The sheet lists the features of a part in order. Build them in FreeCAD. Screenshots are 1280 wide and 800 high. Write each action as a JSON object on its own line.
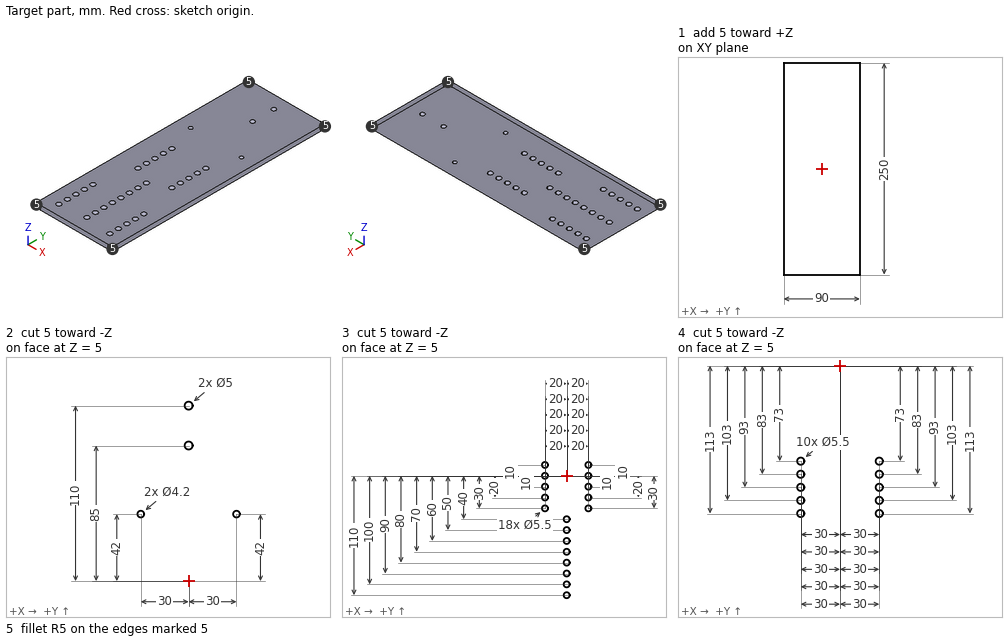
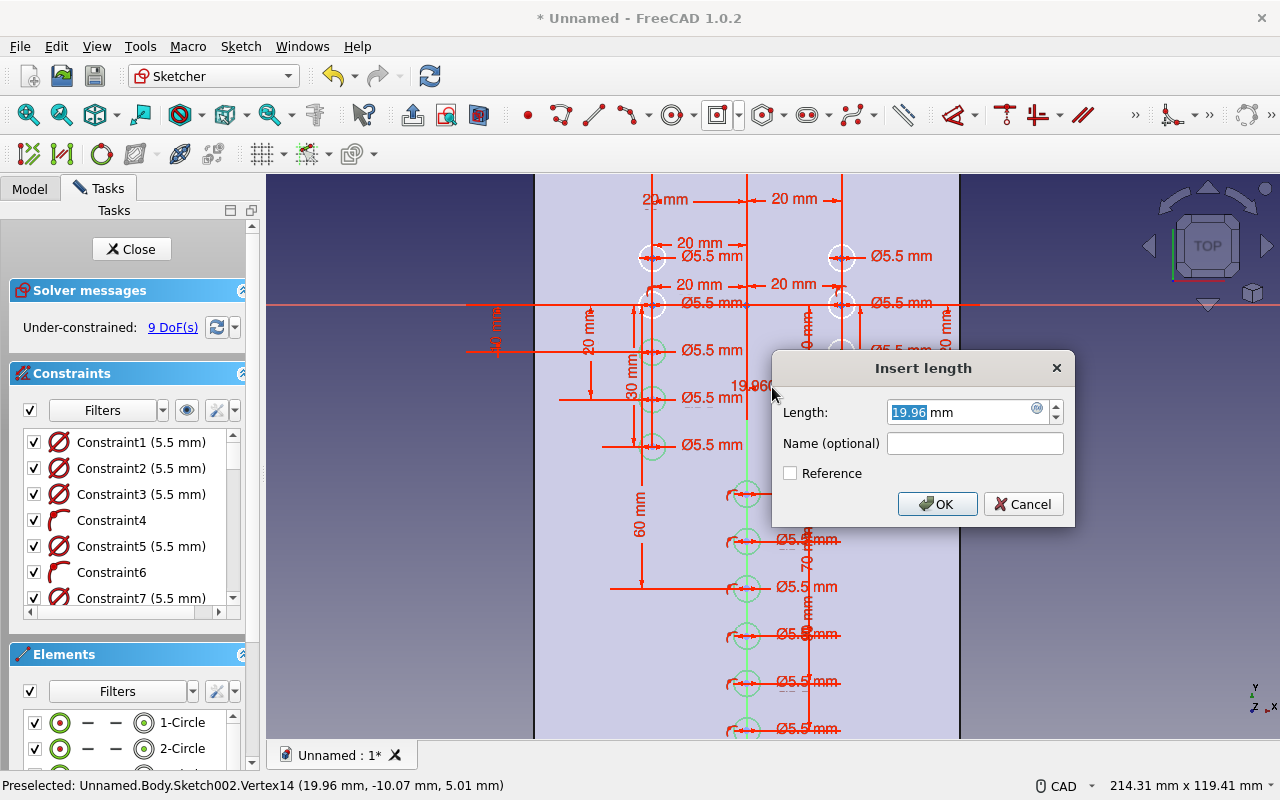
{"action": "type", "text": "20"}
{"action": "key", "text": "Return"}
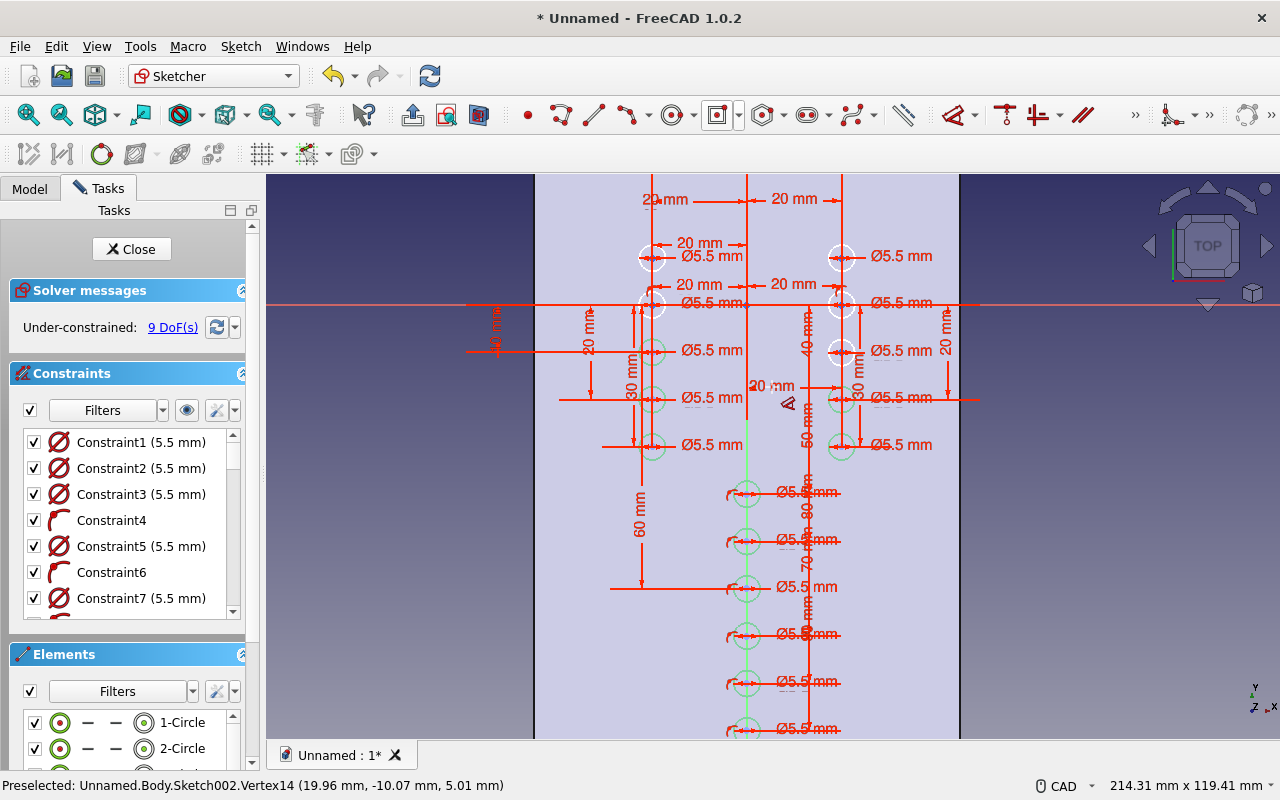
{"action": "left_click", "coordinate": [842, 353]}
{"action": "left_click", "coordinate": [713, 329]}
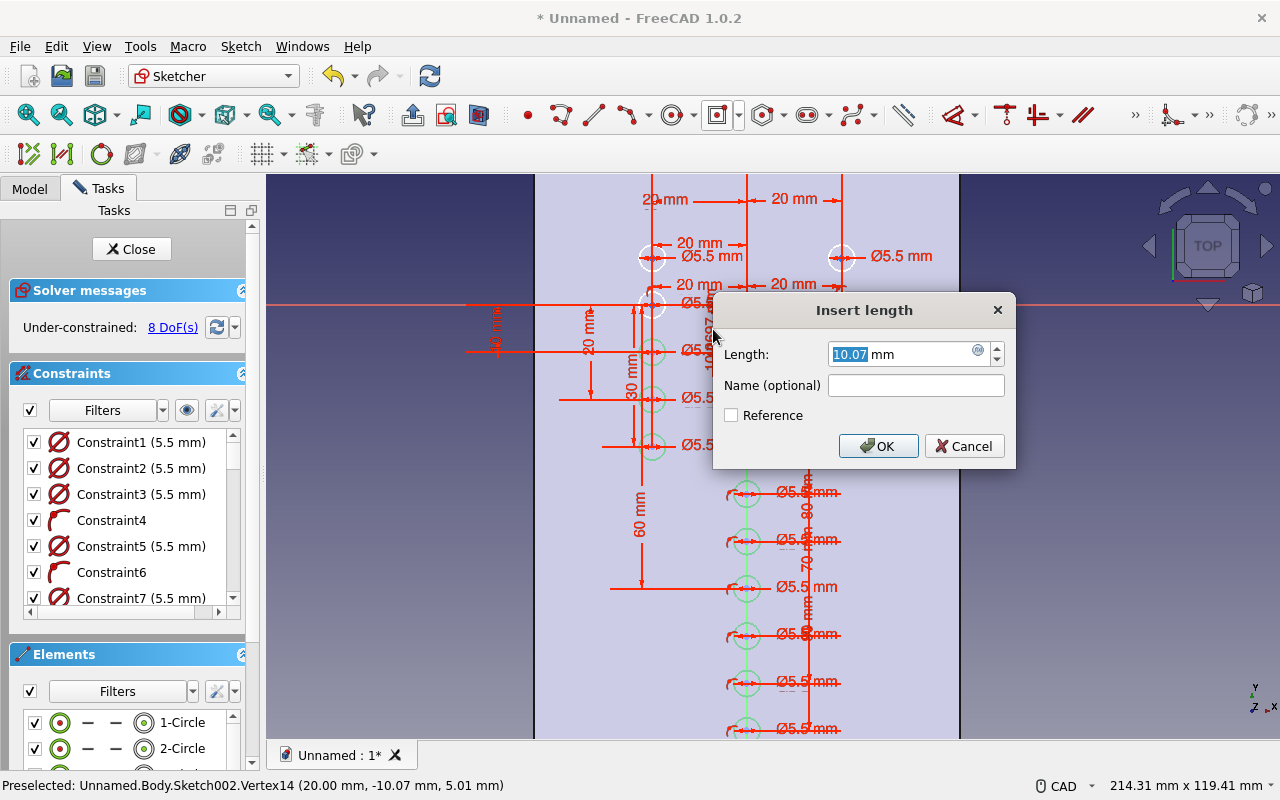
{"action": "type", "text": "10"}
{"action": "key", "text": "Return"}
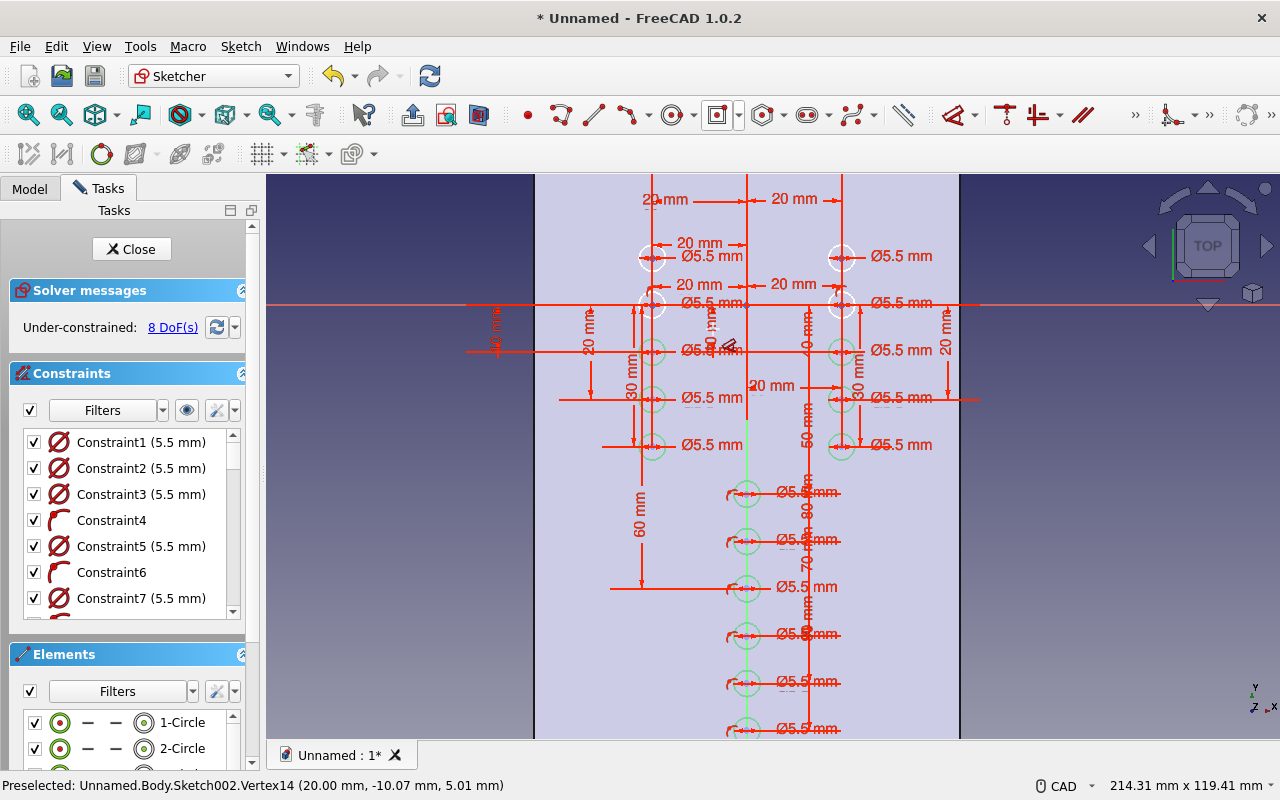
{"action": "left_click", "coordinate": [652, 305]}
{"action": "left_click", "coordinate": [721, 363]}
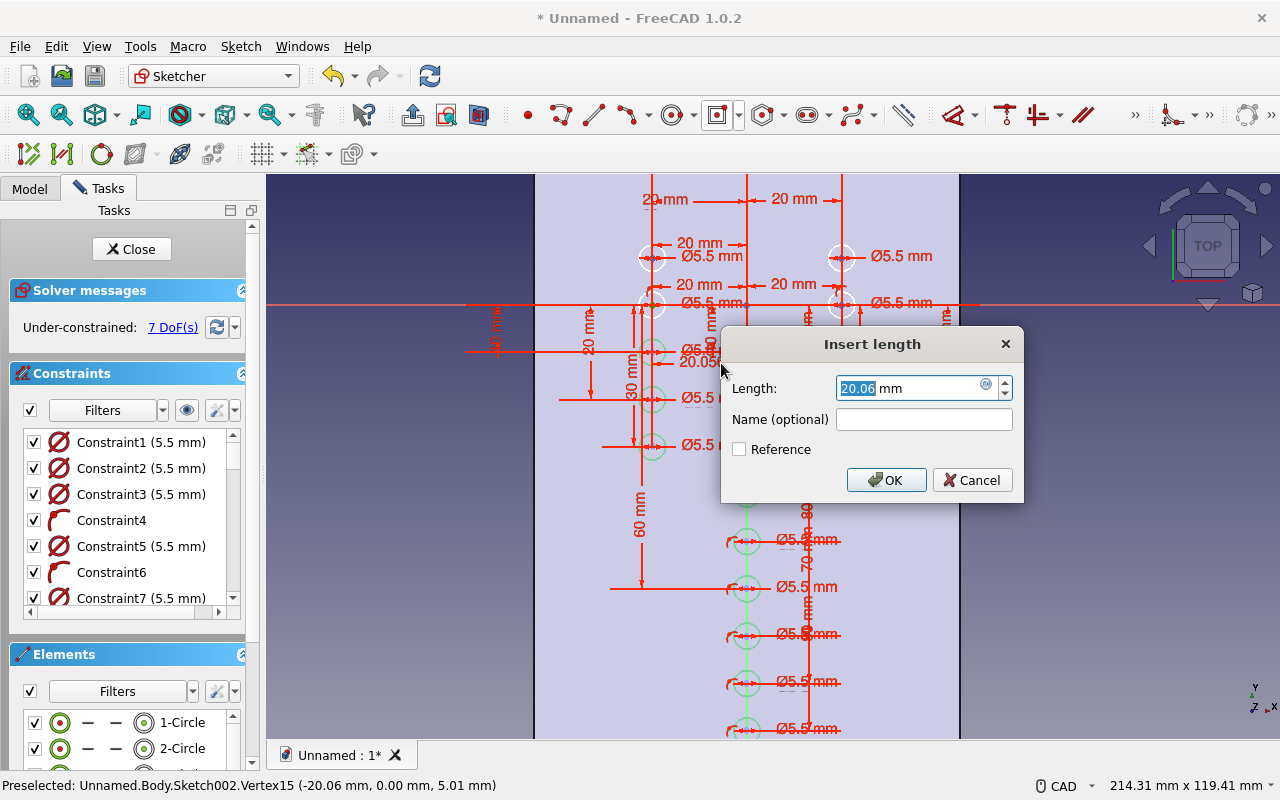
{"action": "type", "text": "20"}
{"action": "key", "text": "Return"}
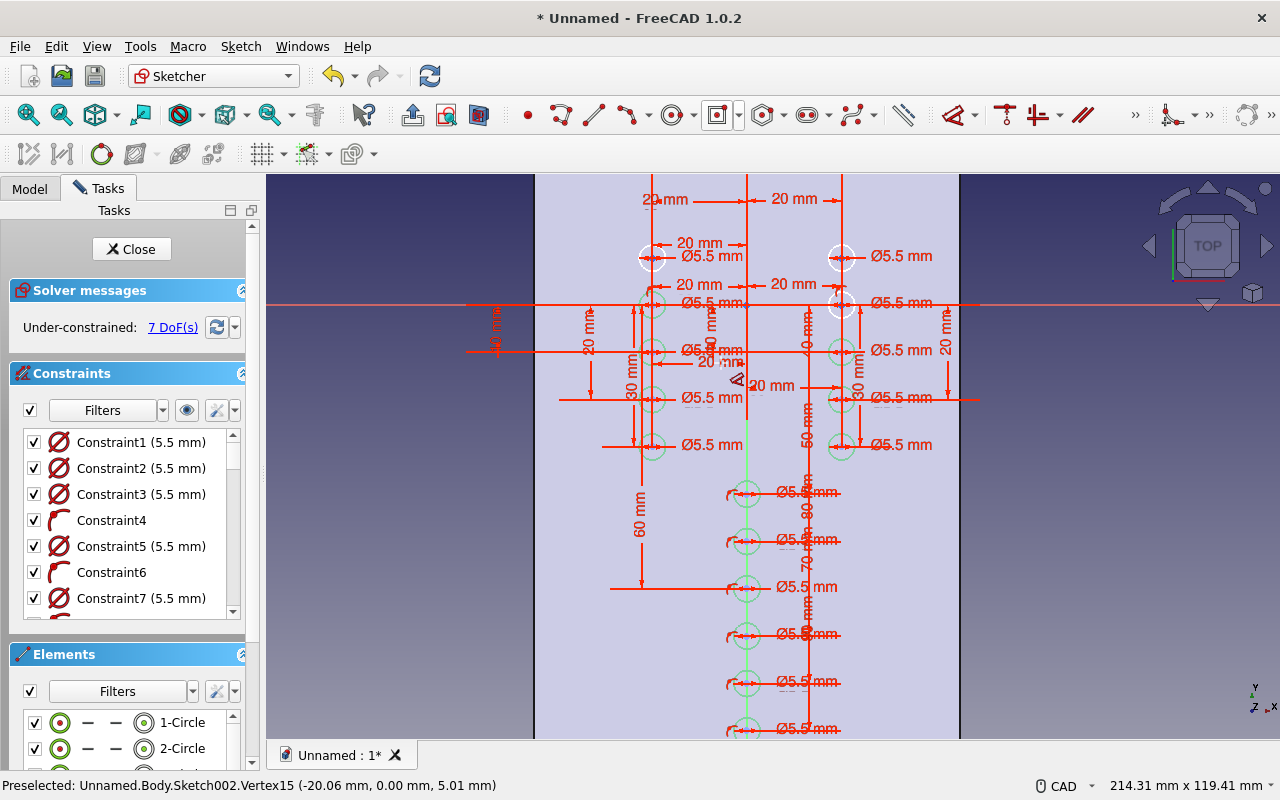
{"action": "left_click", "coordinate": [842, 305]}
{"action": "left_click", "coordinate": [794, 247]}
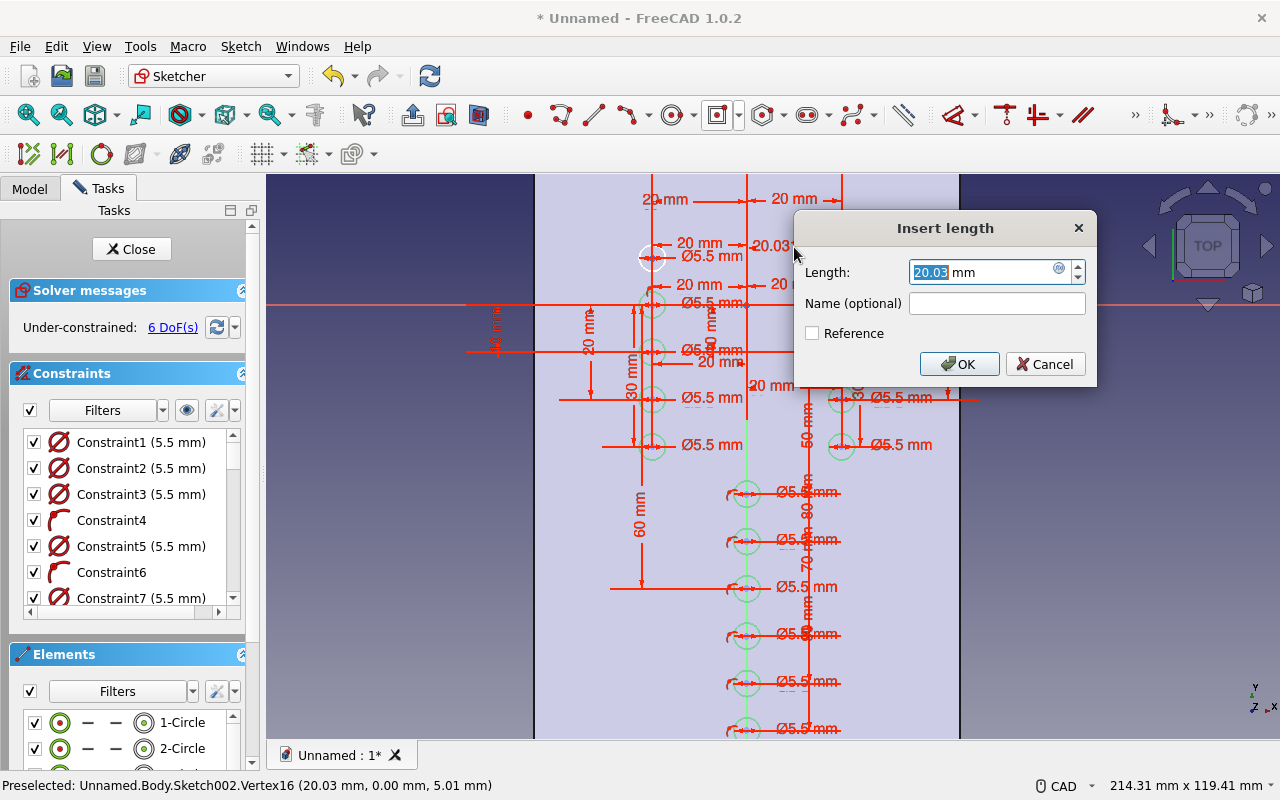
{"action": "type", "text": "20"}
{"action": "key", "text": "Return"}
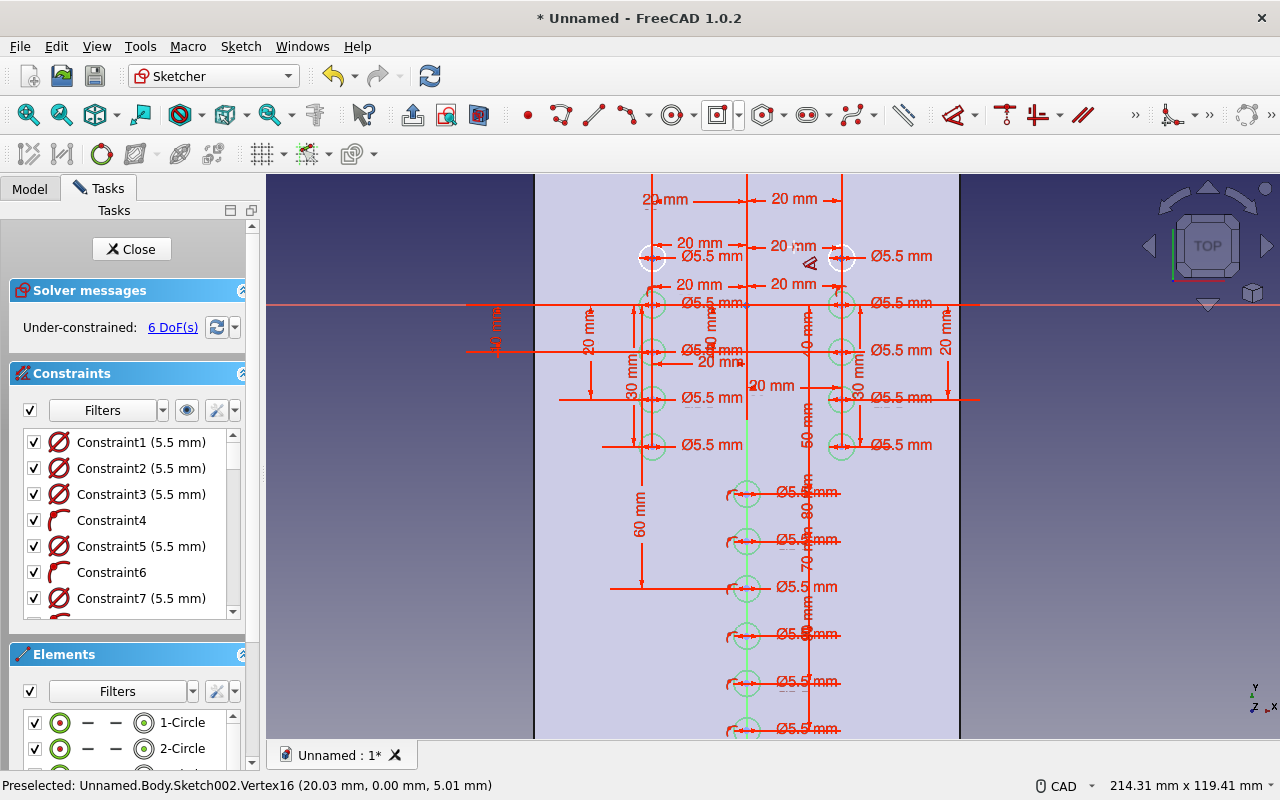
{"action": "left_click", "coordinate": [652, 258]}
{"action": "left_click", "coordinate": [700, 411]}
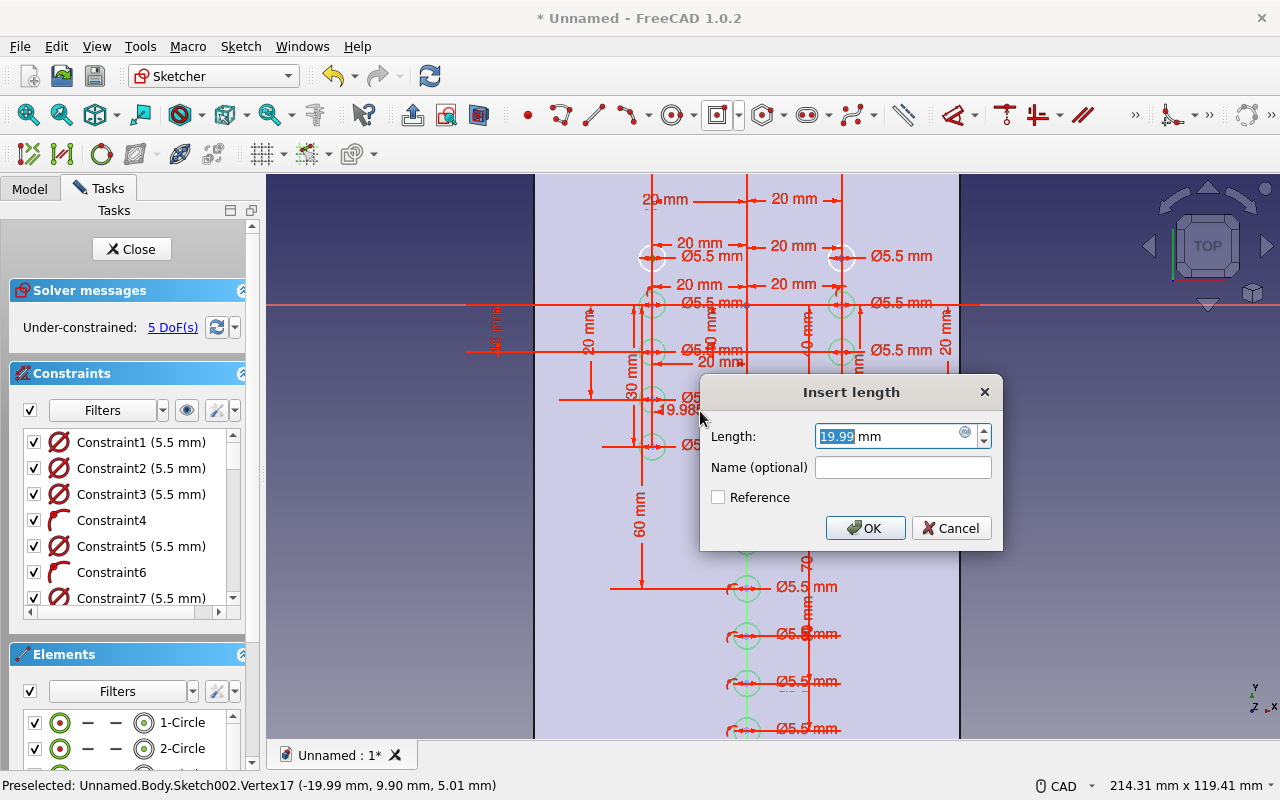
{"action": "type", "text": "20"}
{"action": "key", "text": "Return"}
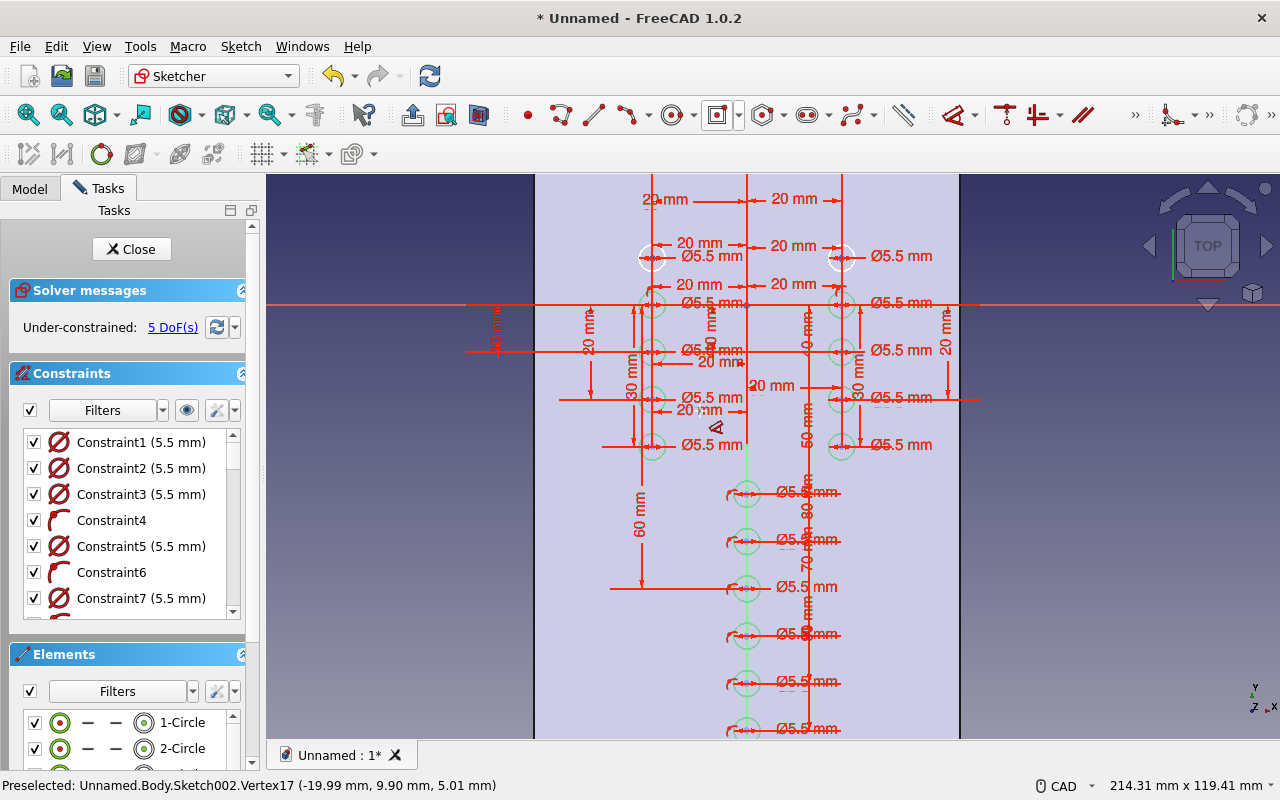
{"action": "left_click", "coordinate": [652, 258]}
{"action": "left_click", "coordinate": [618, 282]}